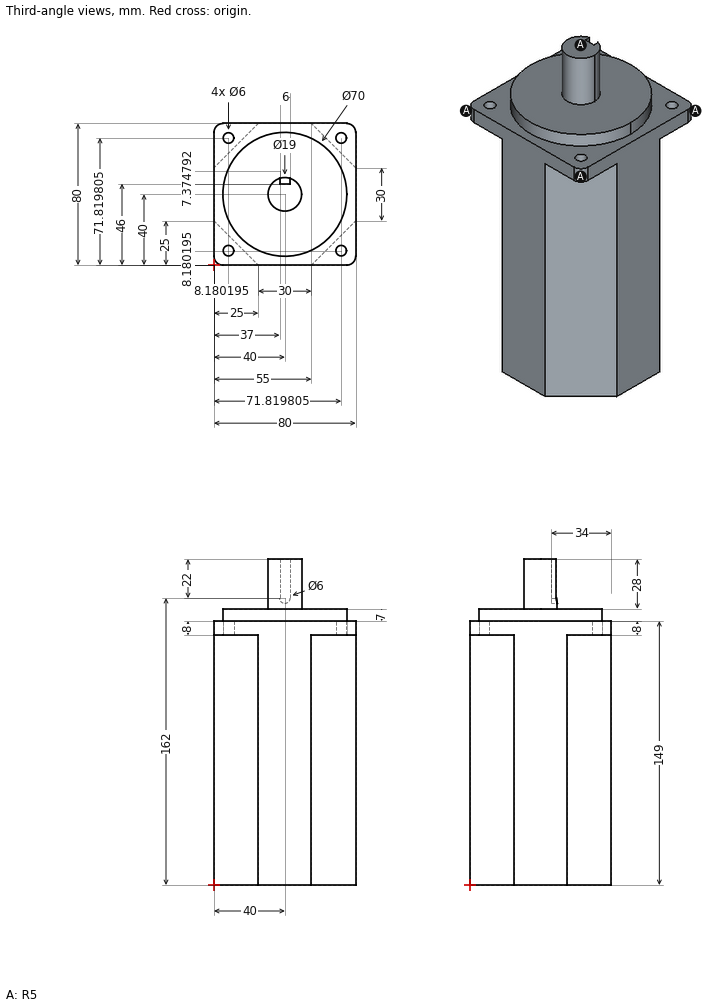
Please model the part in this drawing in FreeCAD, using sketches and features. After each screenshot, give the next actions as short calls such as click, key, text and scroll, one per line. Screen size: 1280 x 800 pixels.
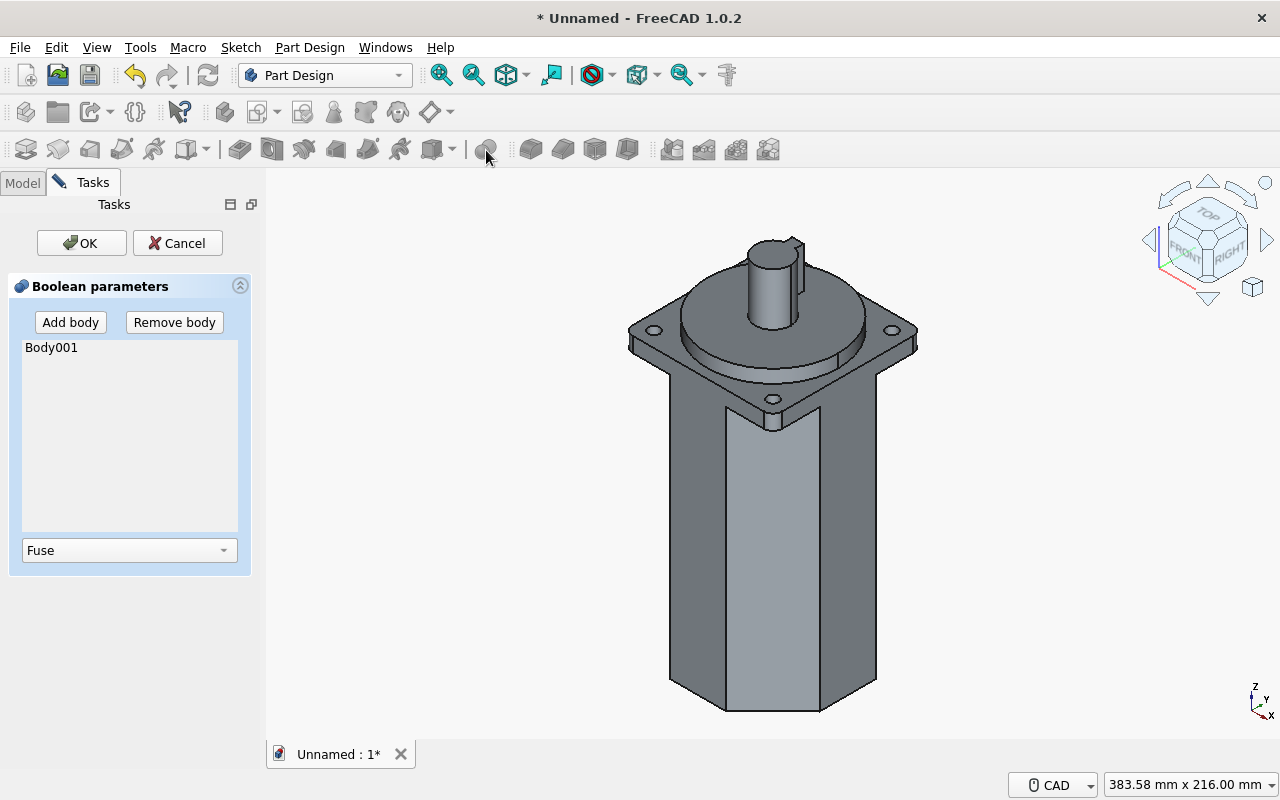
click(130, 550)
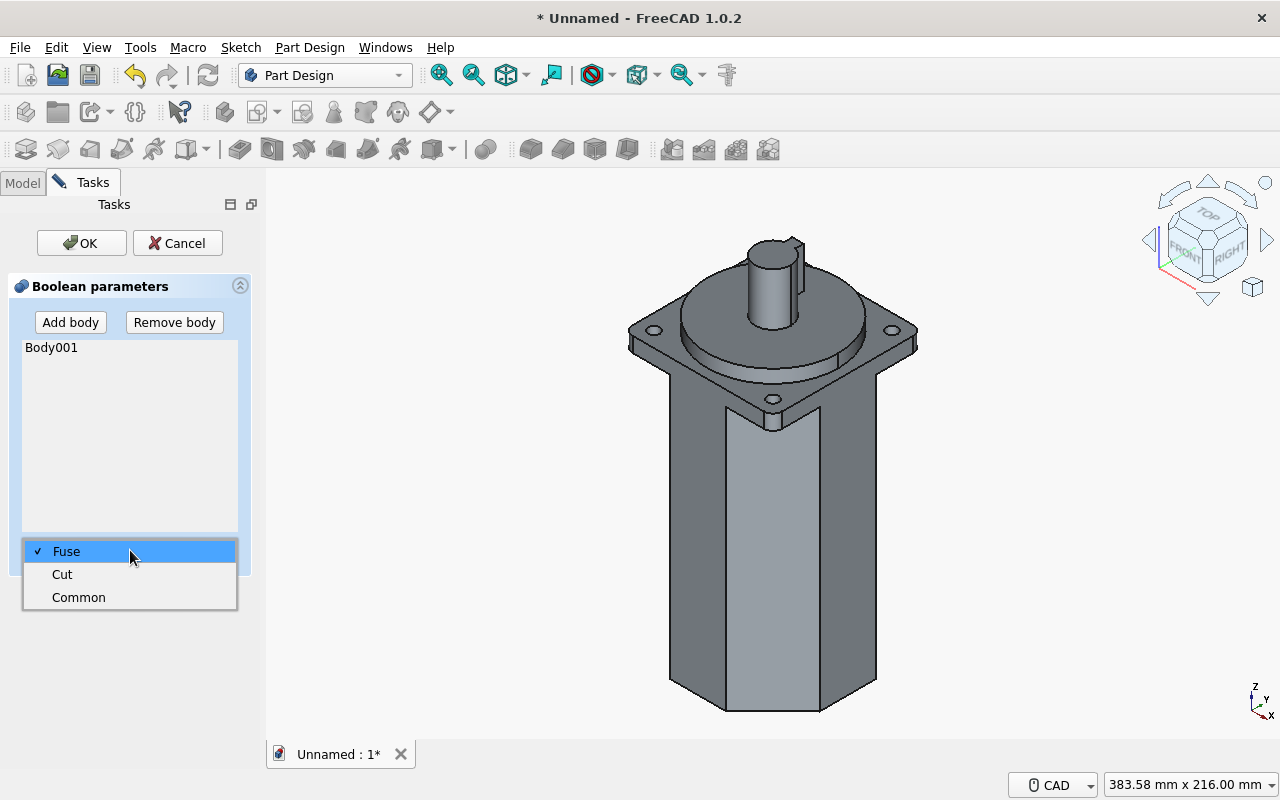
click(129, 574)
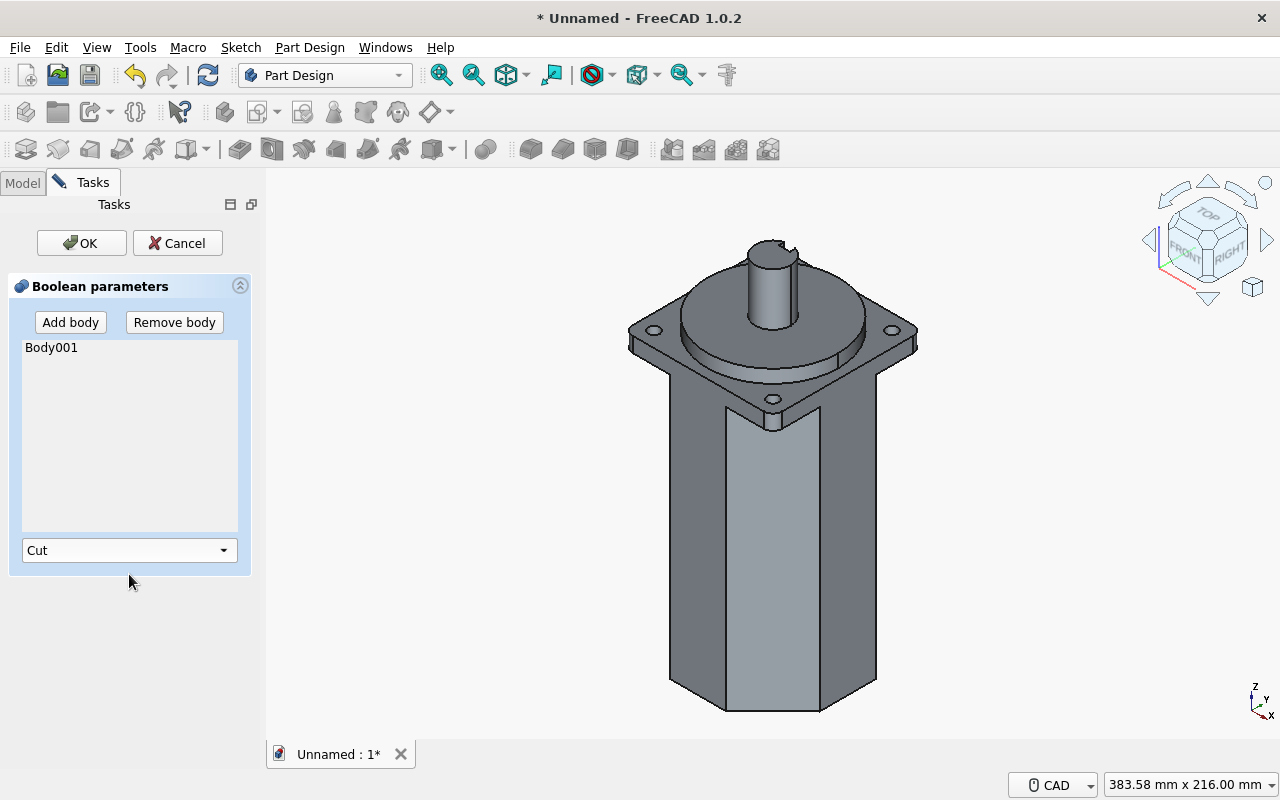
click(82, 243)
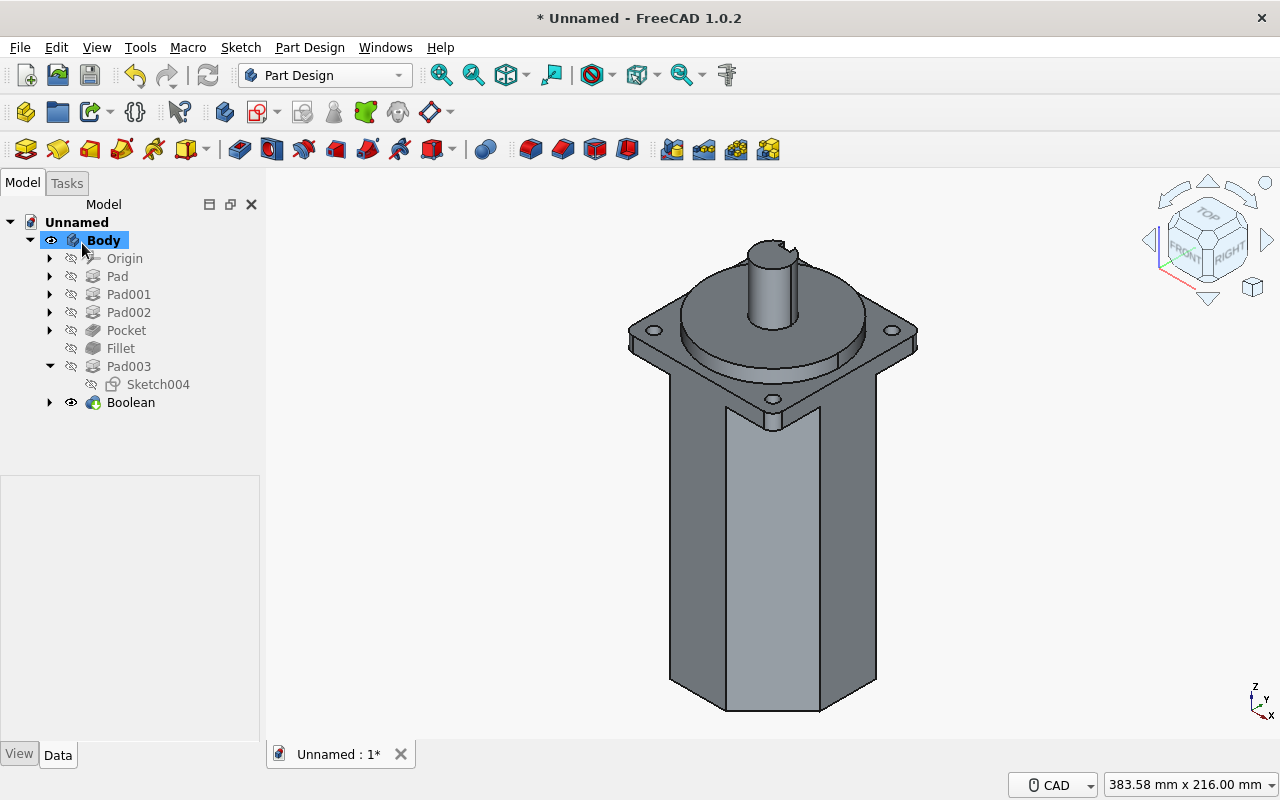
key(4)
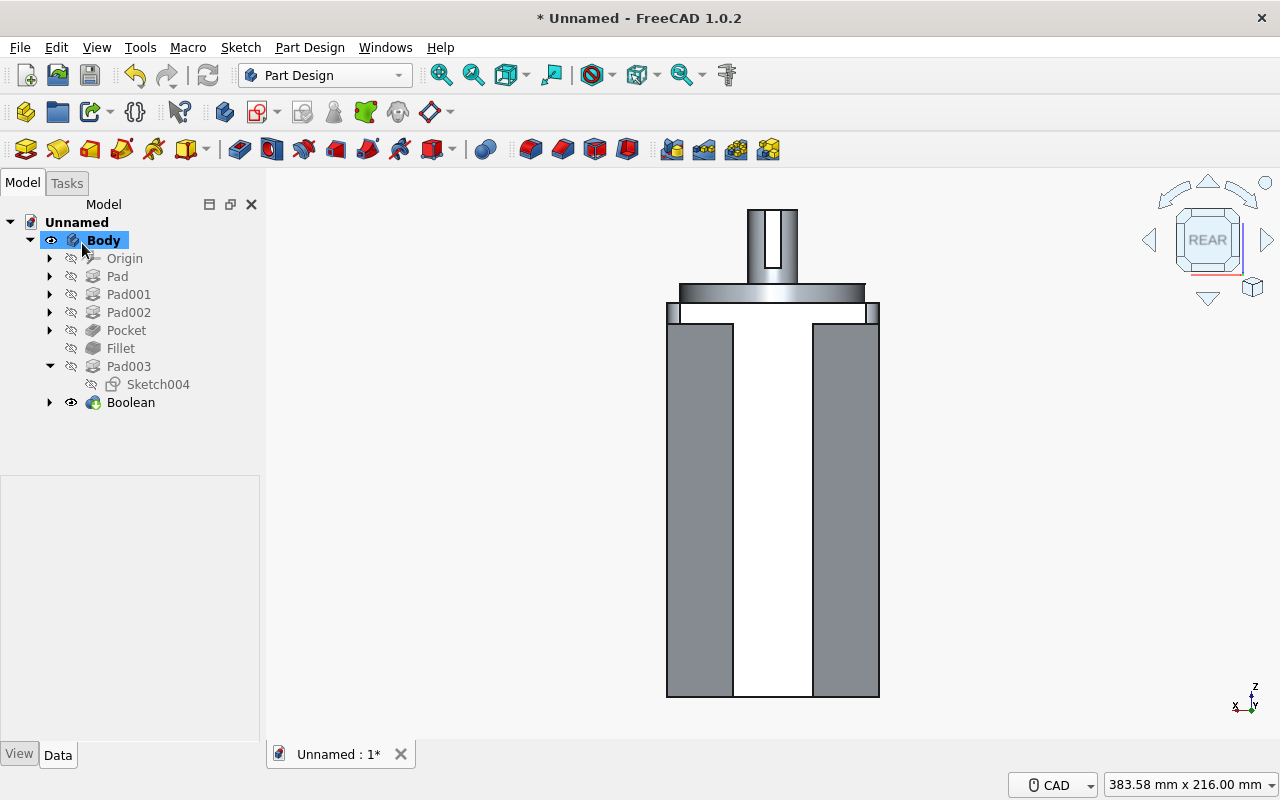
click(773, 386)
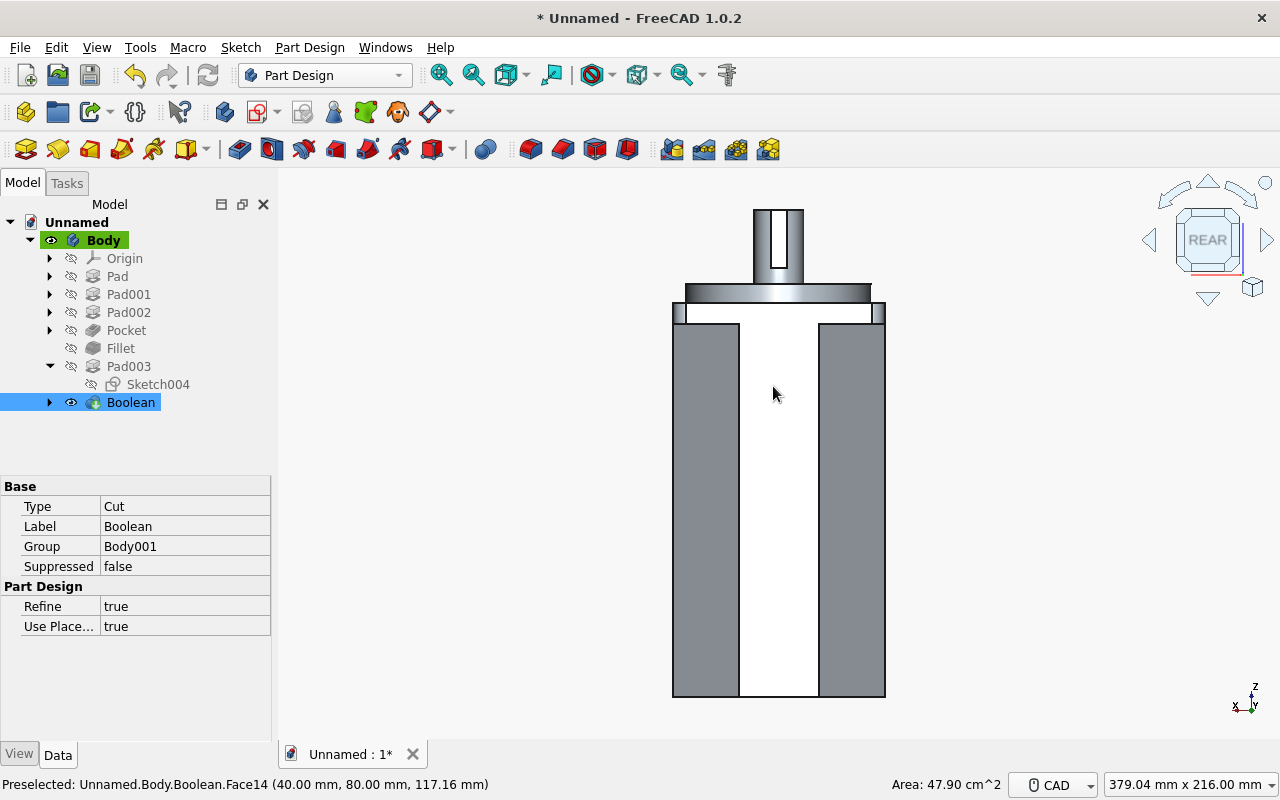
click(258, 112)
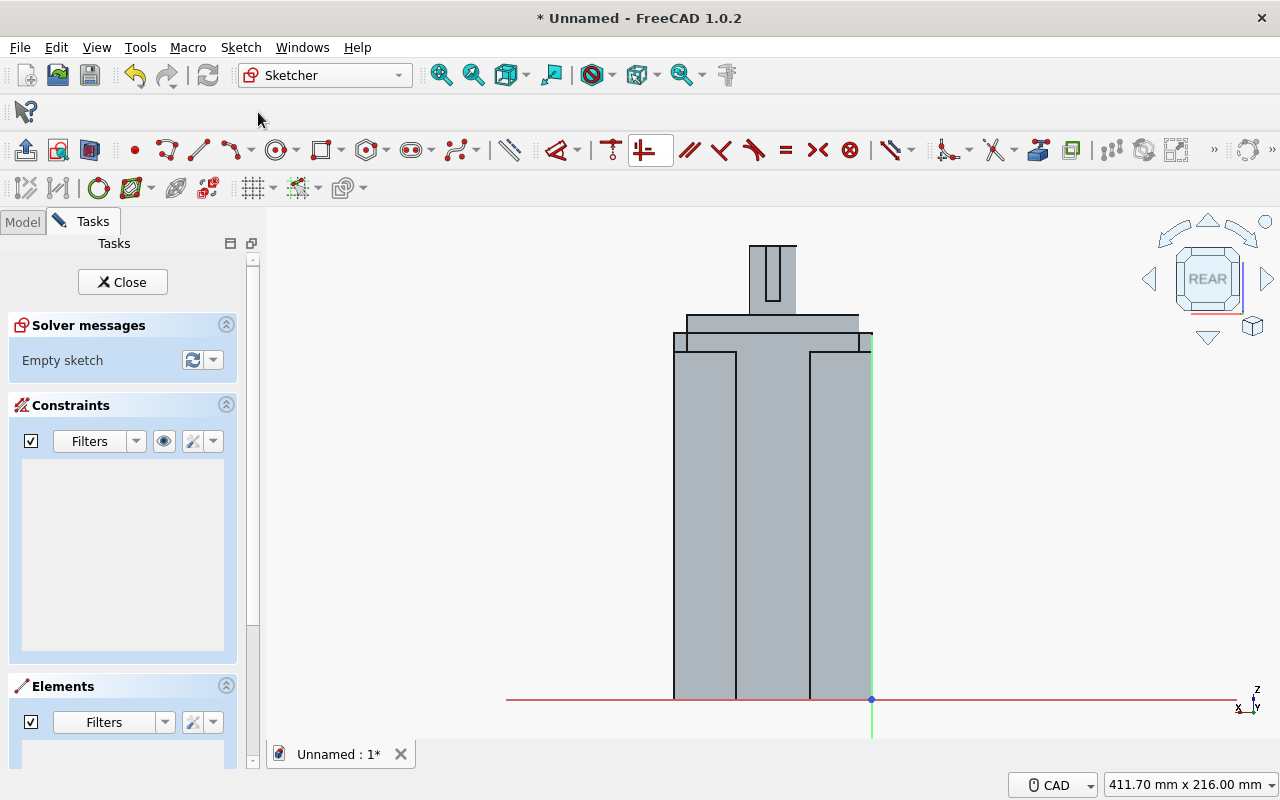
scroll(777, 292, up, 15)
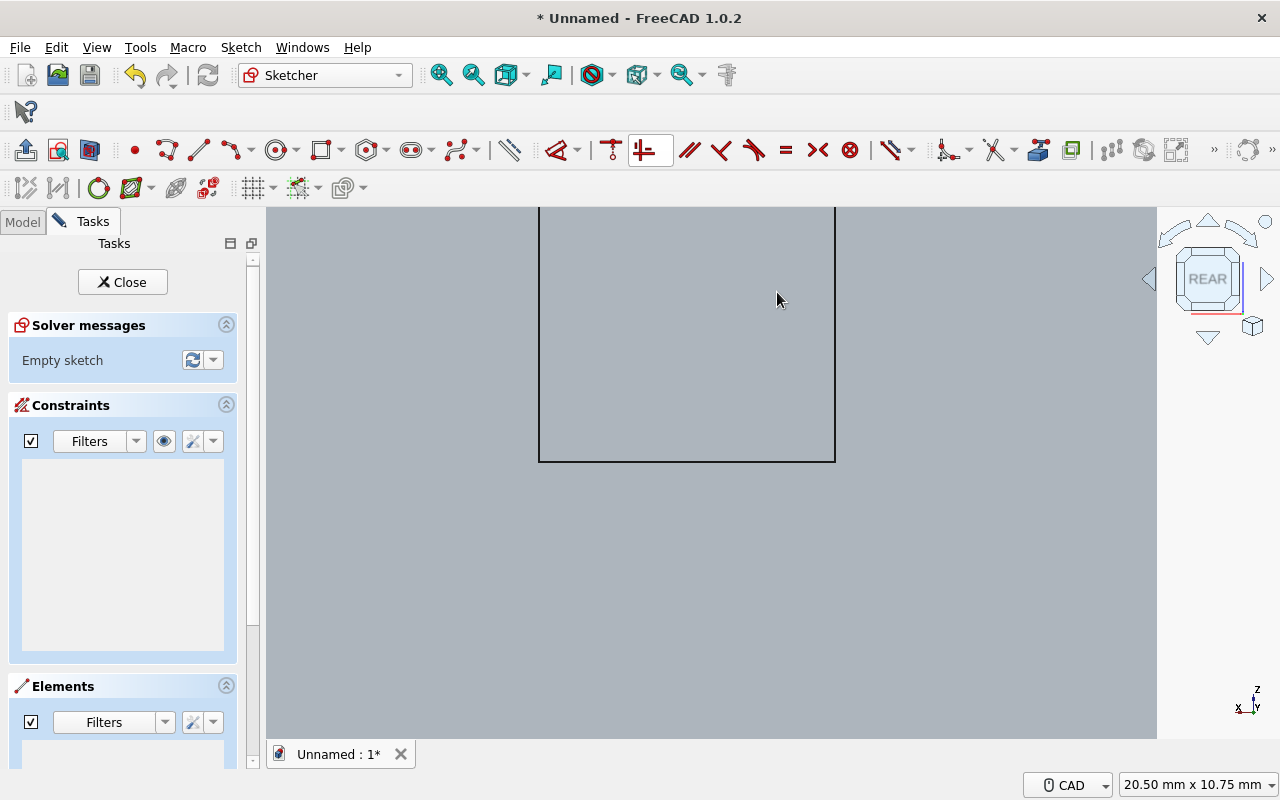
key(g)
key(c)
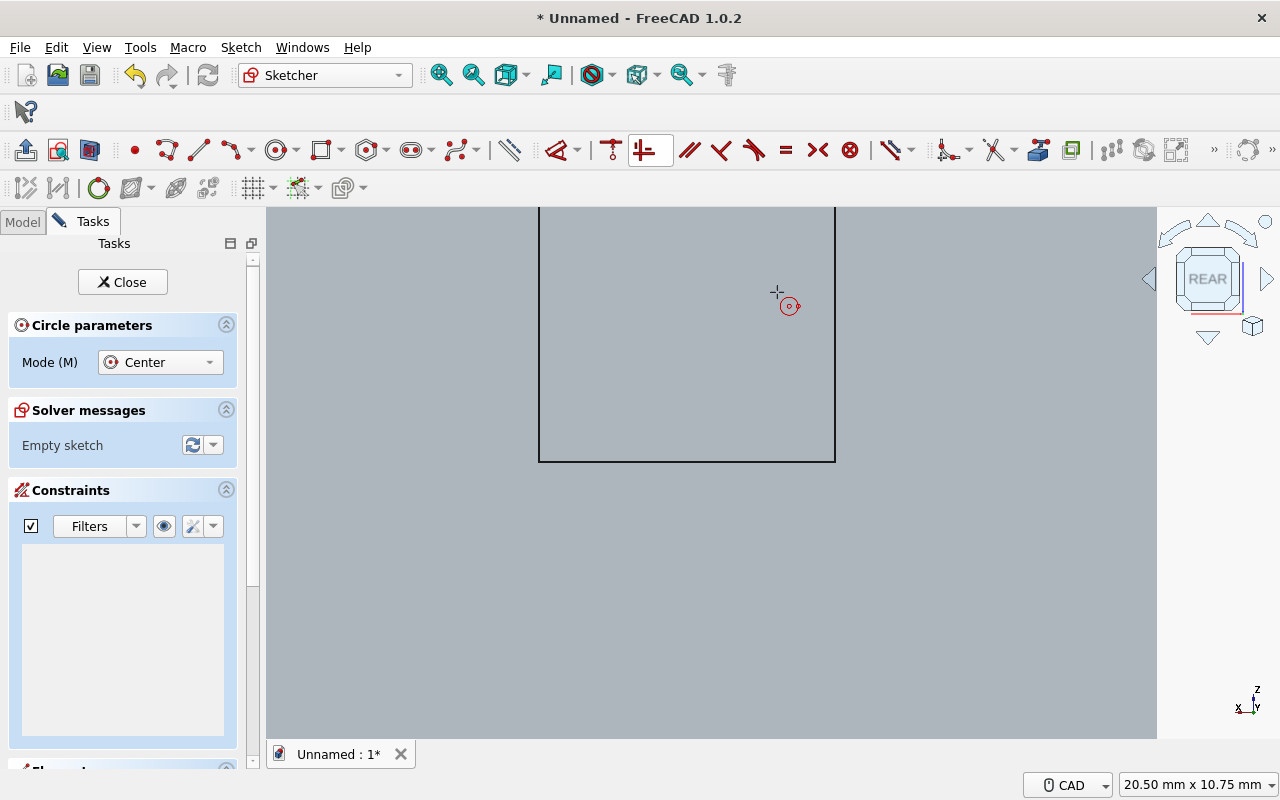
click(687, 462)
click(792, 357)
key(Escape)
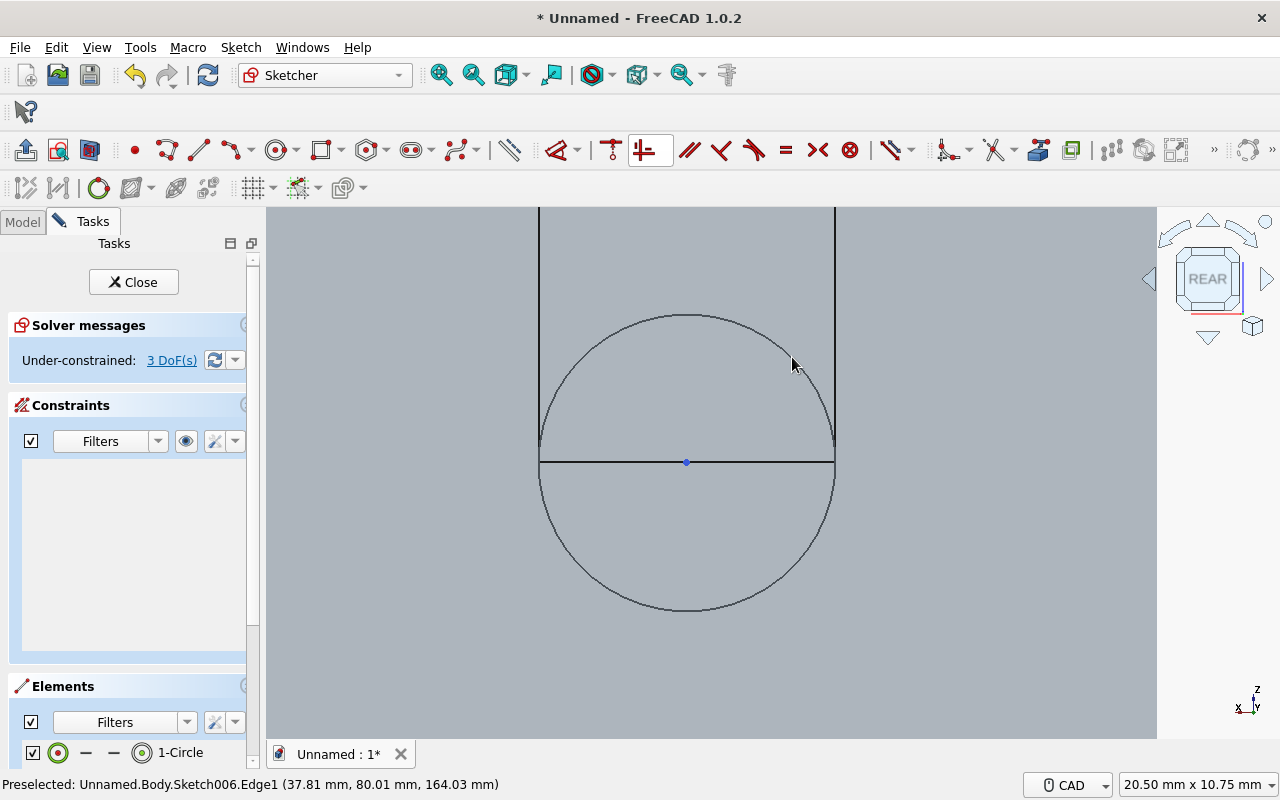
key(d)